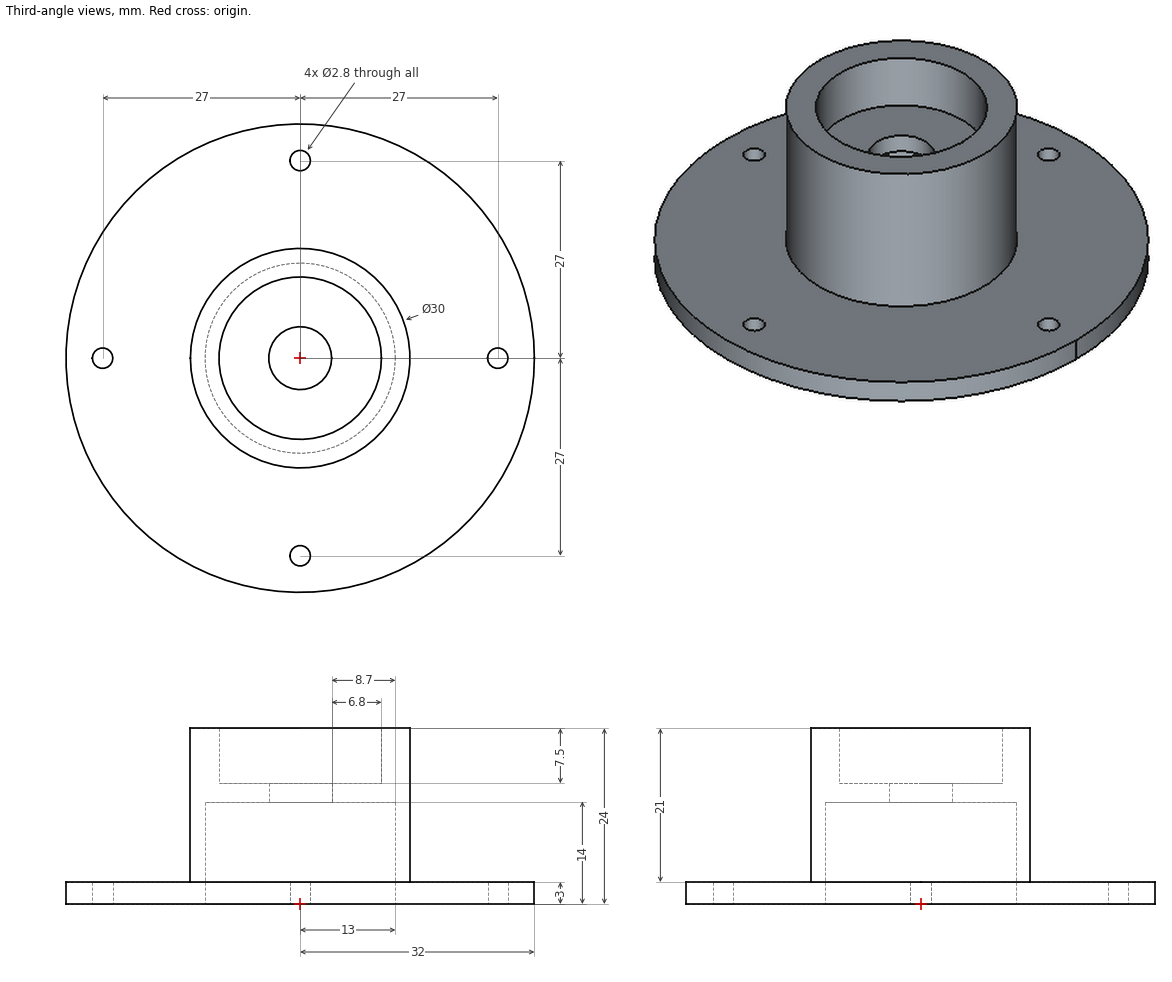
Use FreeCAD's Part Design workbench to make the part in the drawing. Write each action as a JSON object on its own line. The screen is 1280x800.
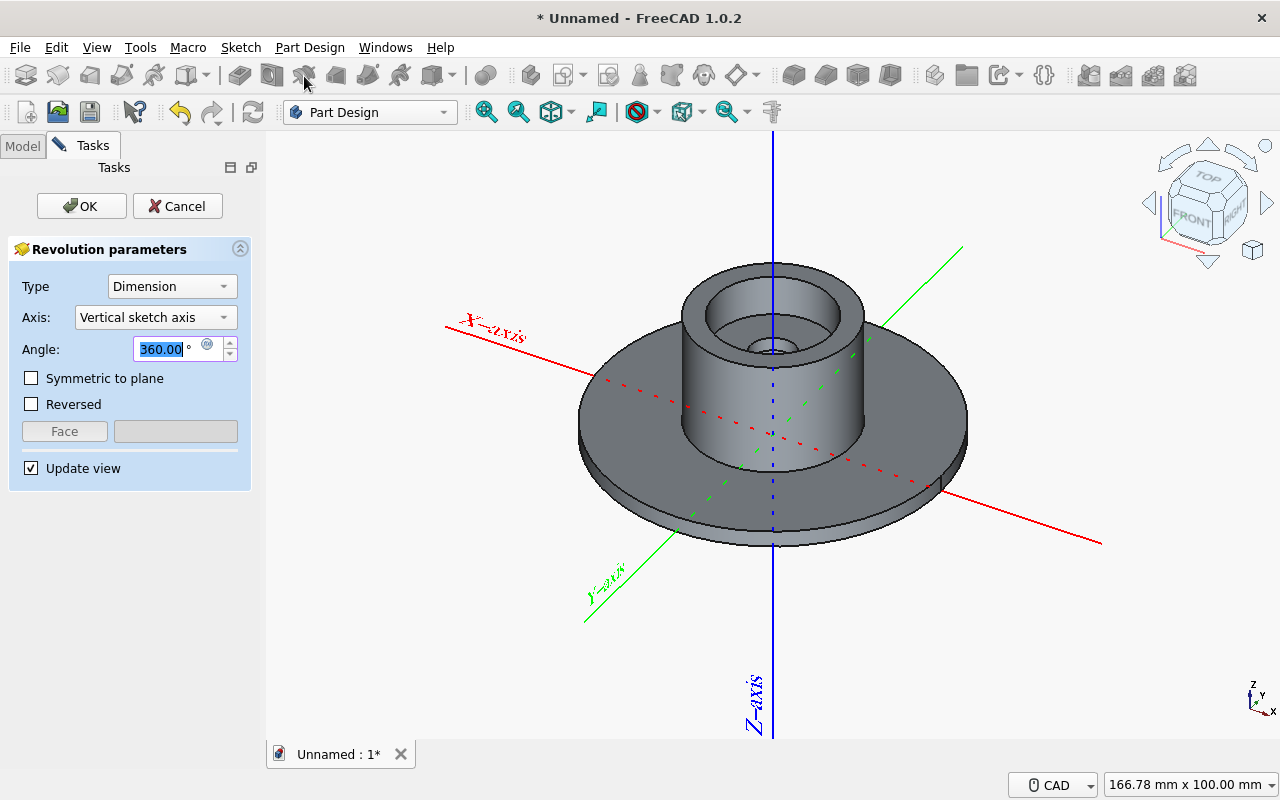
{"action": "left_click", "coordinate": [82, 206]}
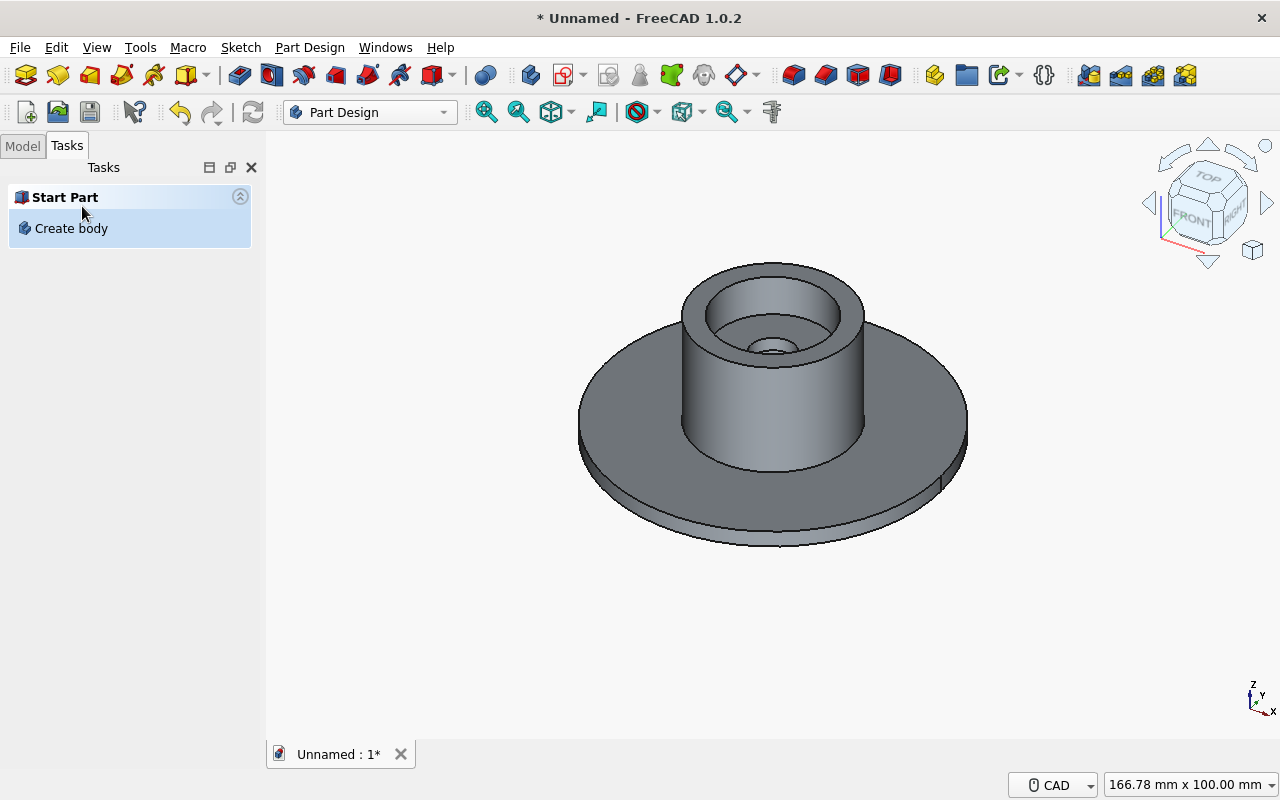
{"action": "left_click", "coordinate": [925, 396]}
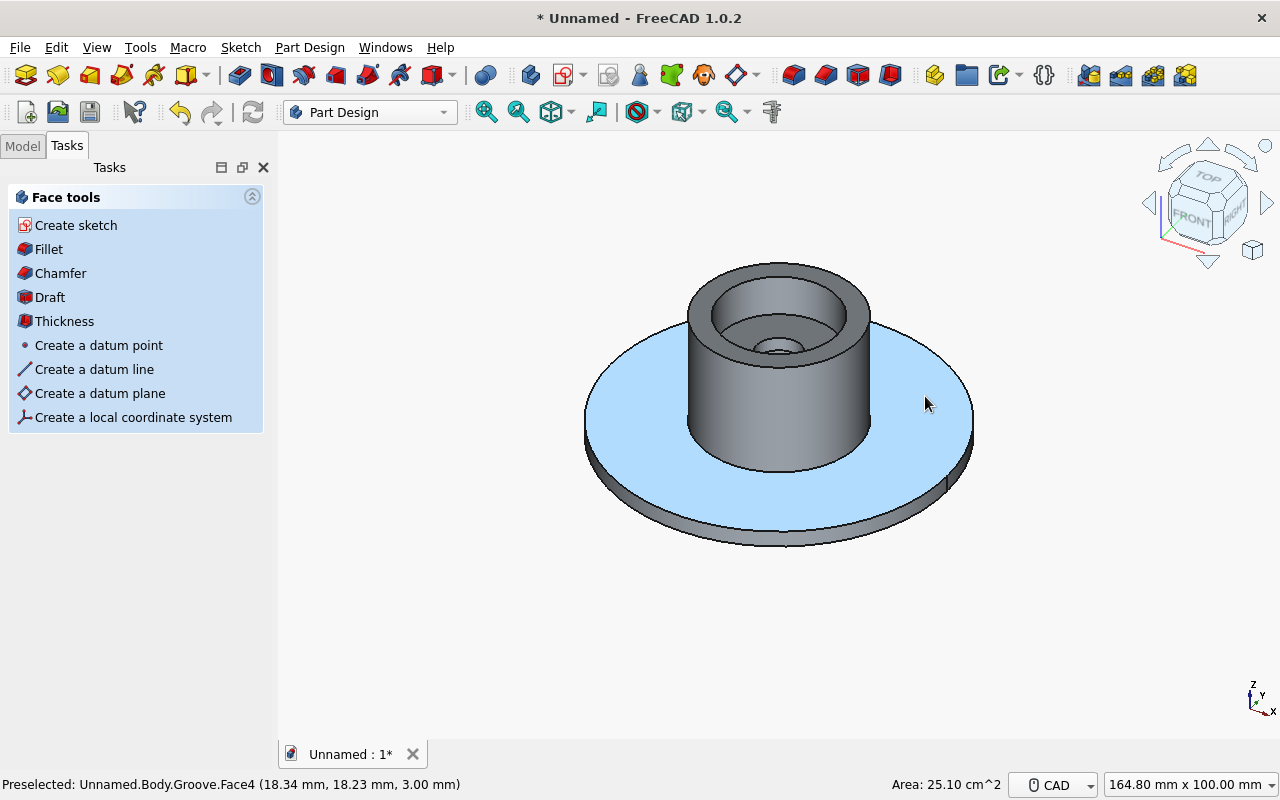
{"action": "left_click", "coordinate": [564, 76]}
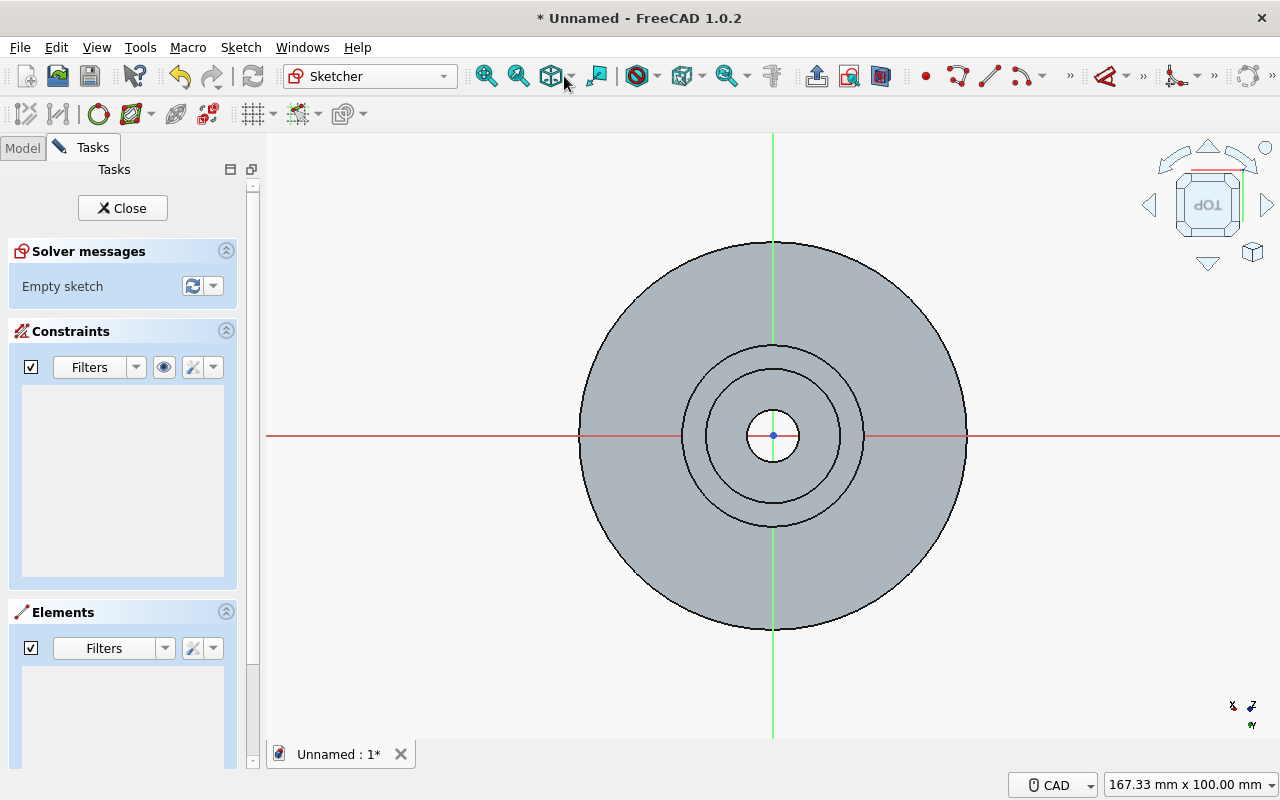
{"action": "left_click", "coordinate": [882, 76]}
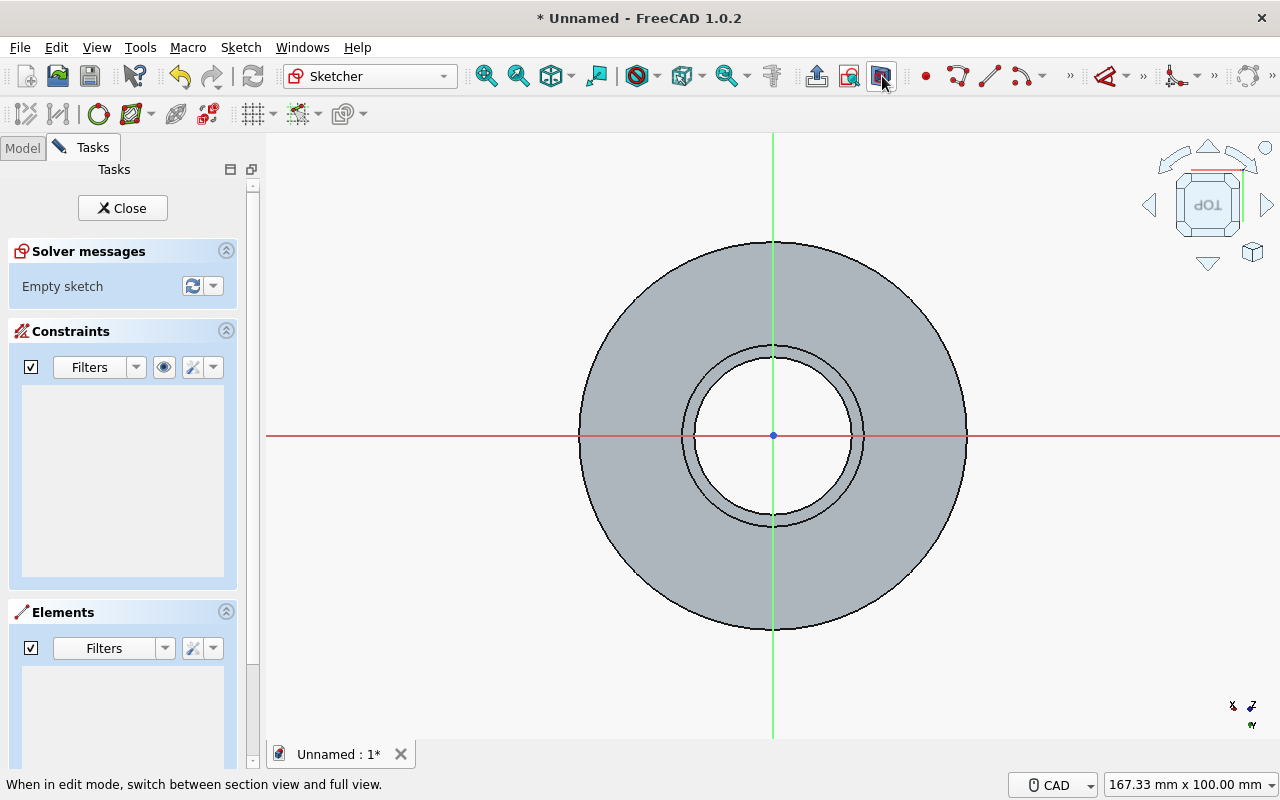
{"action": "key", "text": "g c"}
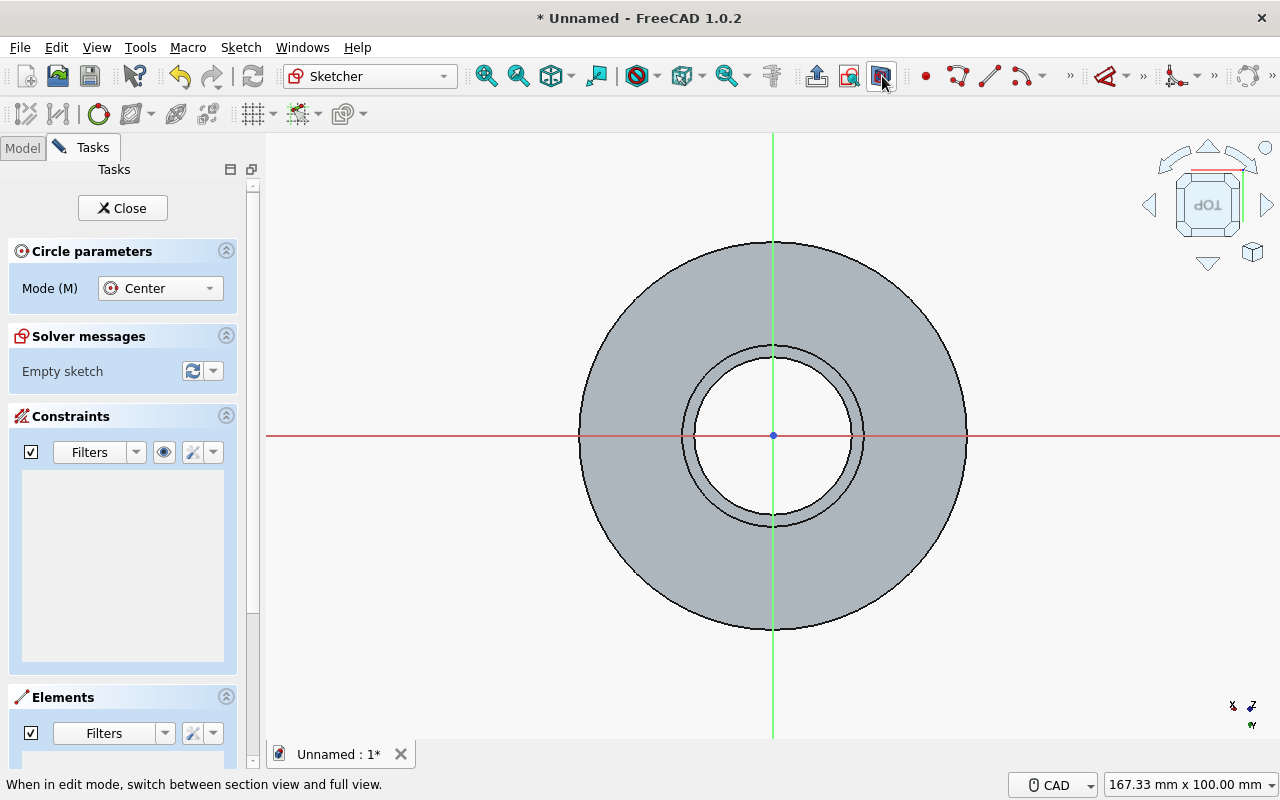
{"action": "scroll", "coordinate": [773, 600], "scroll_direction": "up", "scroll_amount": 5}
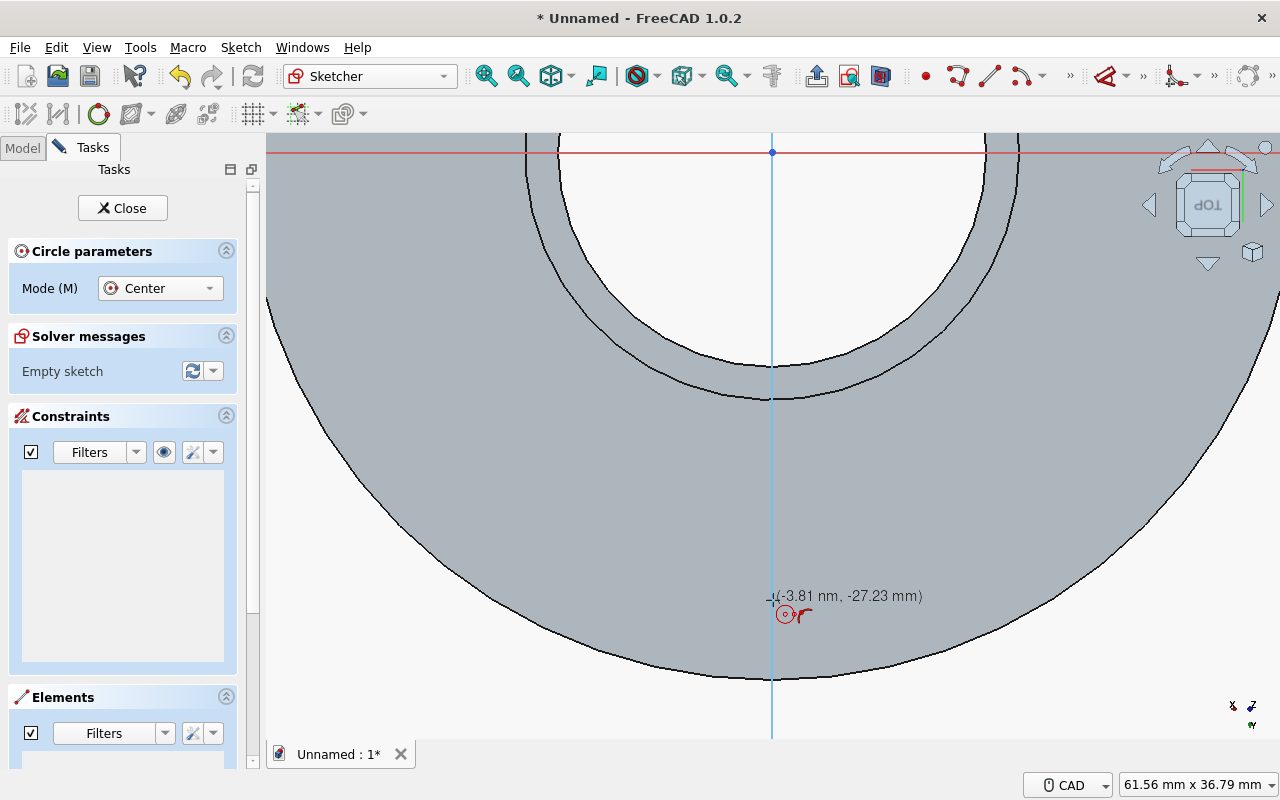
{"action": "left_click", "coordinate": [772, 598]}
{"action": "mouse_move", "coordinate": [788, 581]}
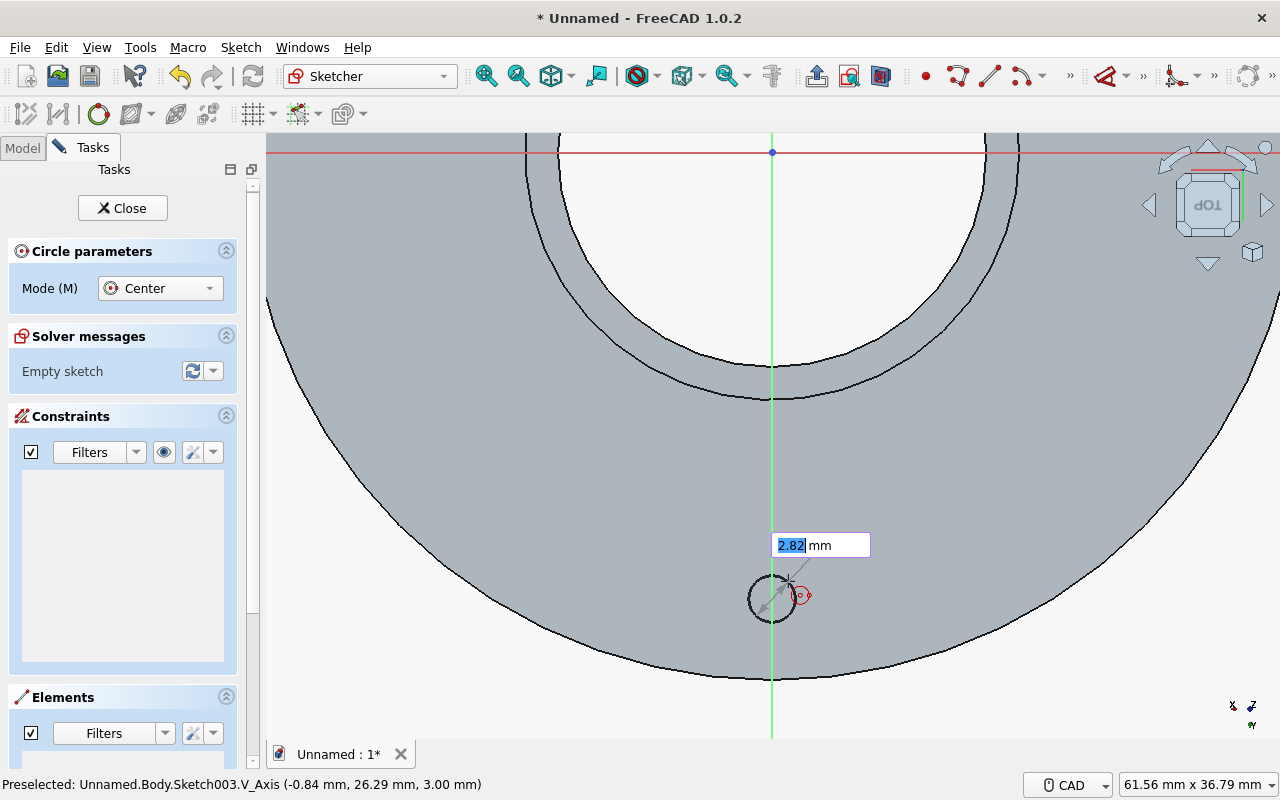
{"action": "type", "text": "2.8"}
{"action": "key", "text": "Return"}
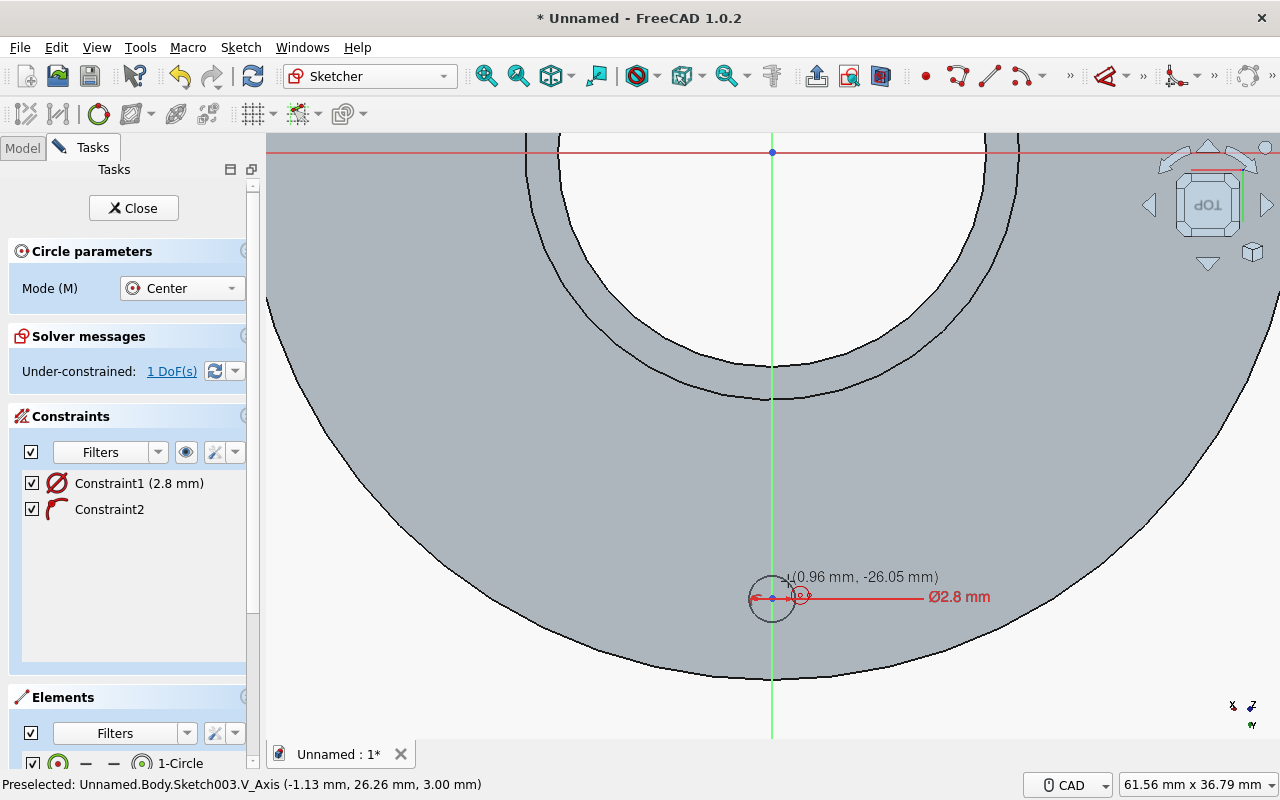
{"action": "scroll", "coordinate": [649, 667], "scroll_direction": "down", "scroll_amount": 4}